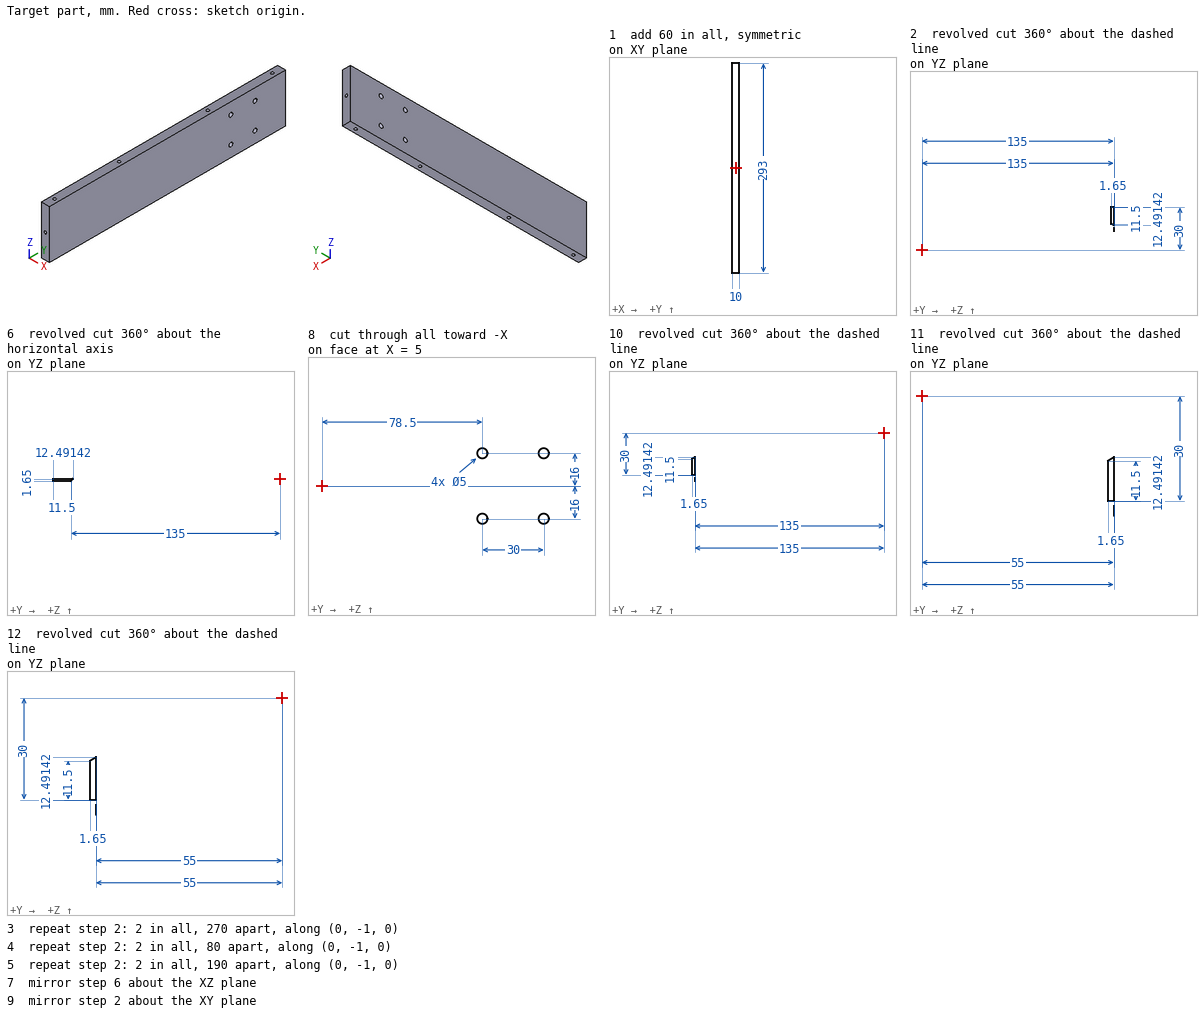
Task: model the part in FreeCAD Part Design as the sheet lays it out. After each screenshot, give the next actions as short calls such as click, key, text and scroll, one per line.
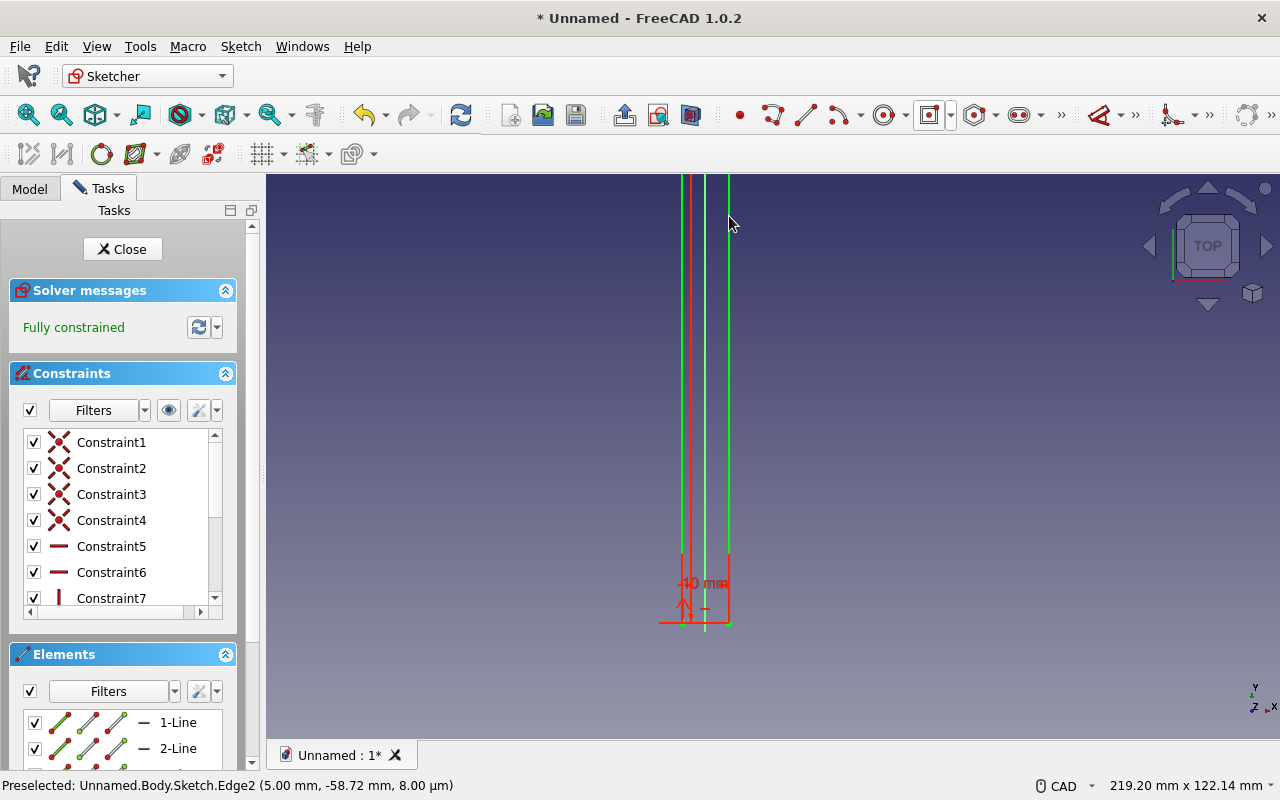
click(123, 249)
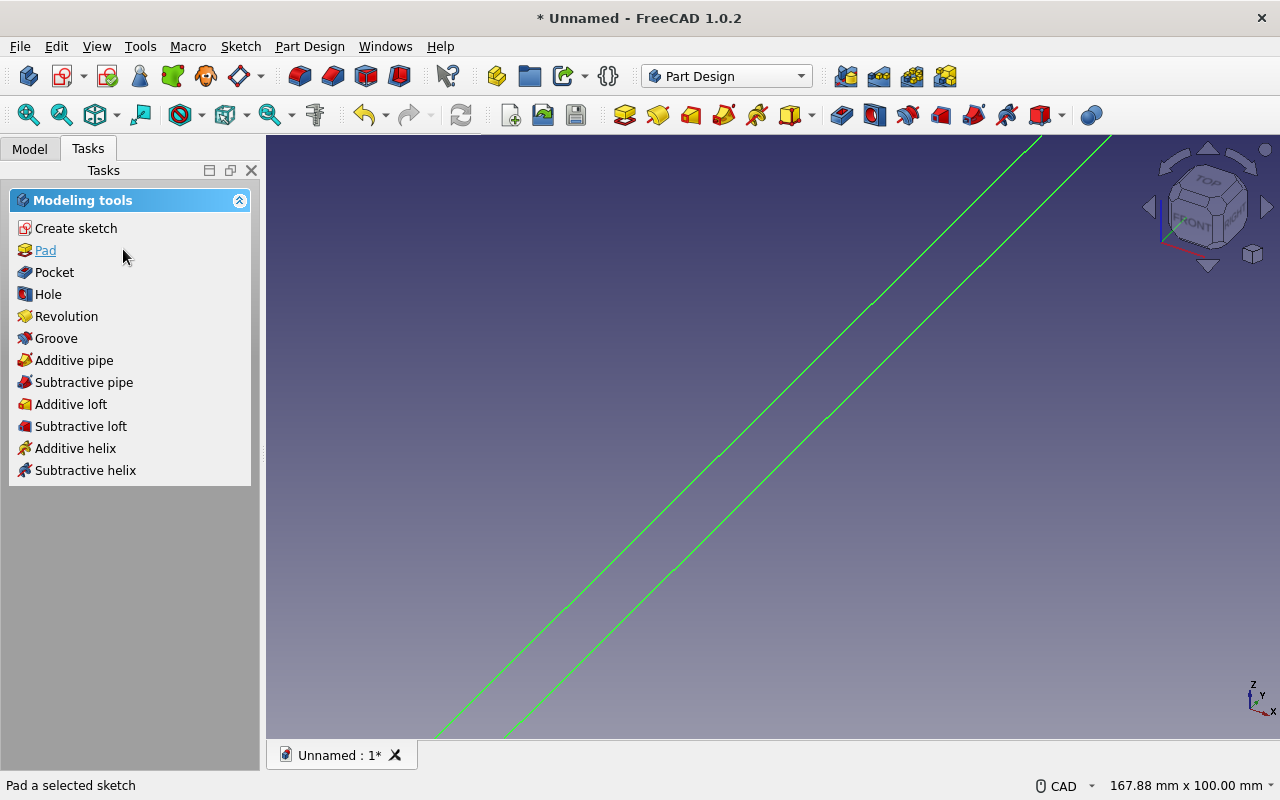
click(625, 116)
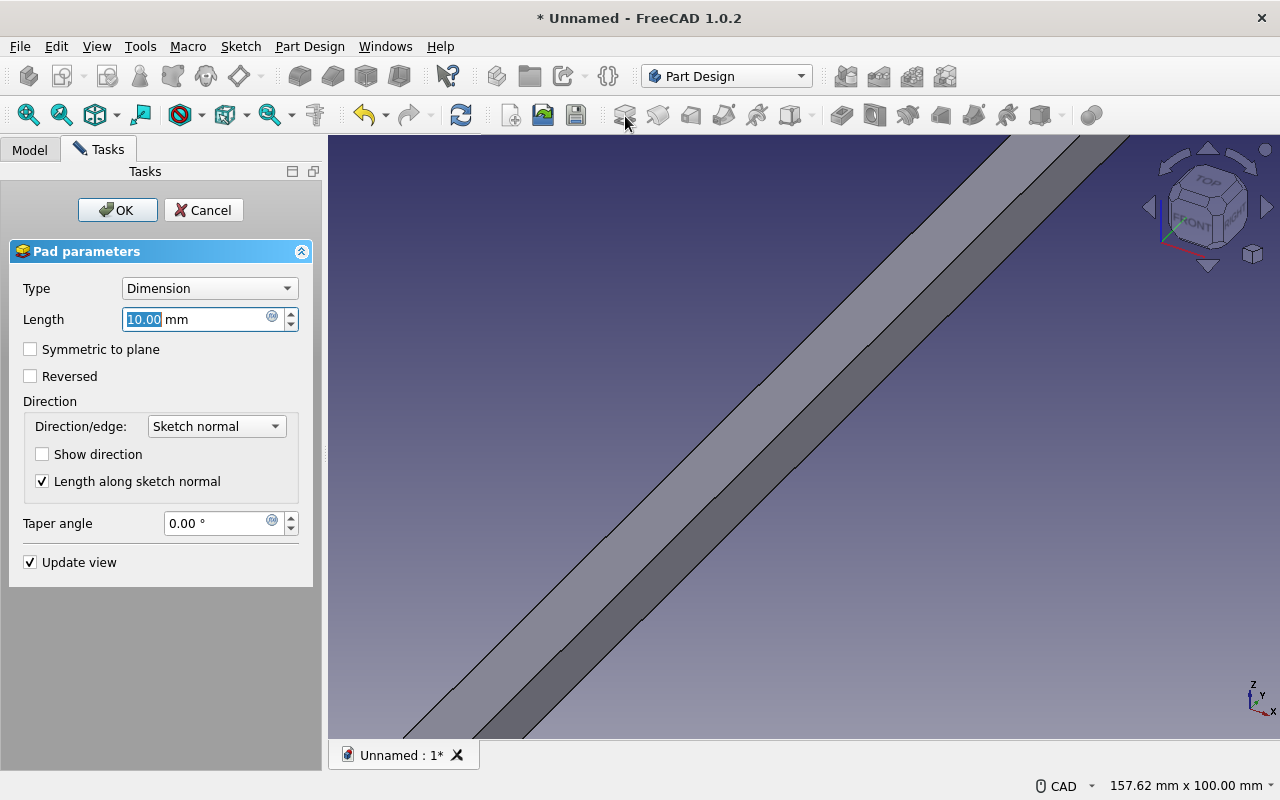
text(60)
key(Tab)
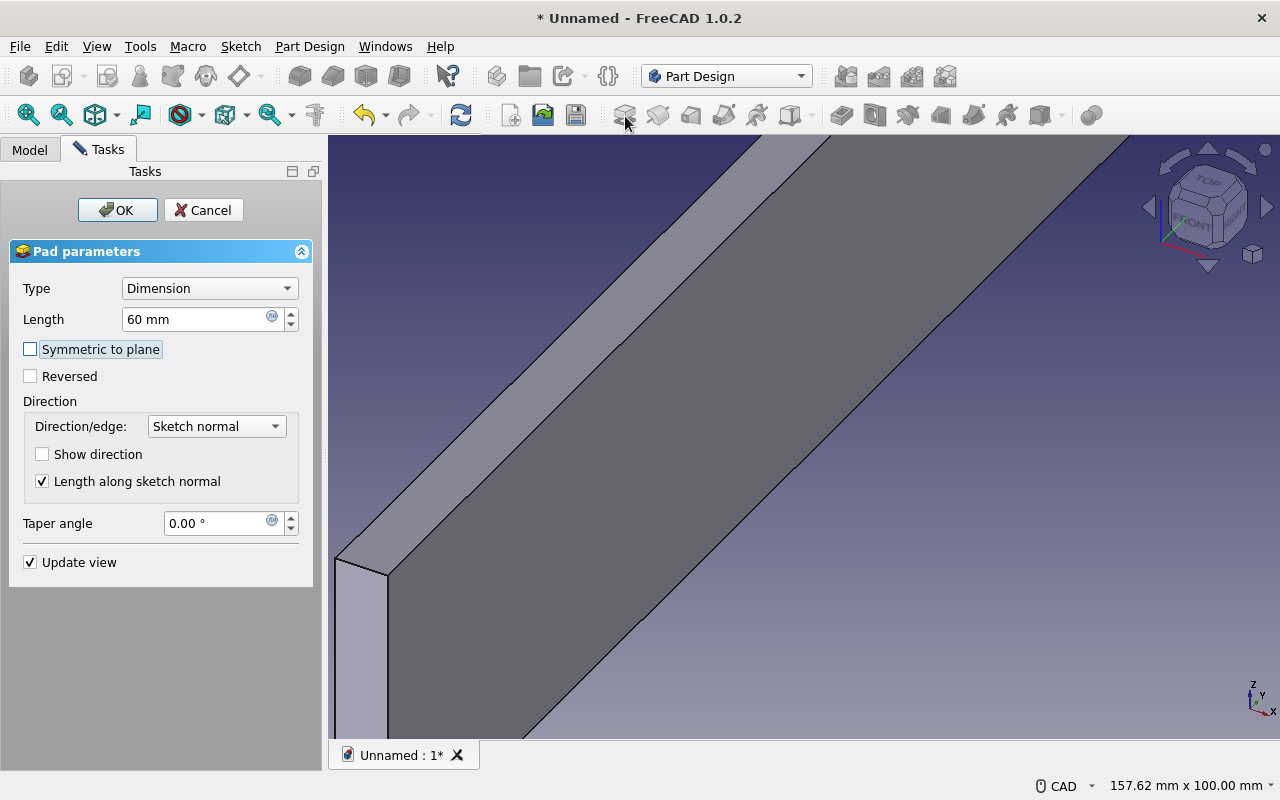
click(31, 349)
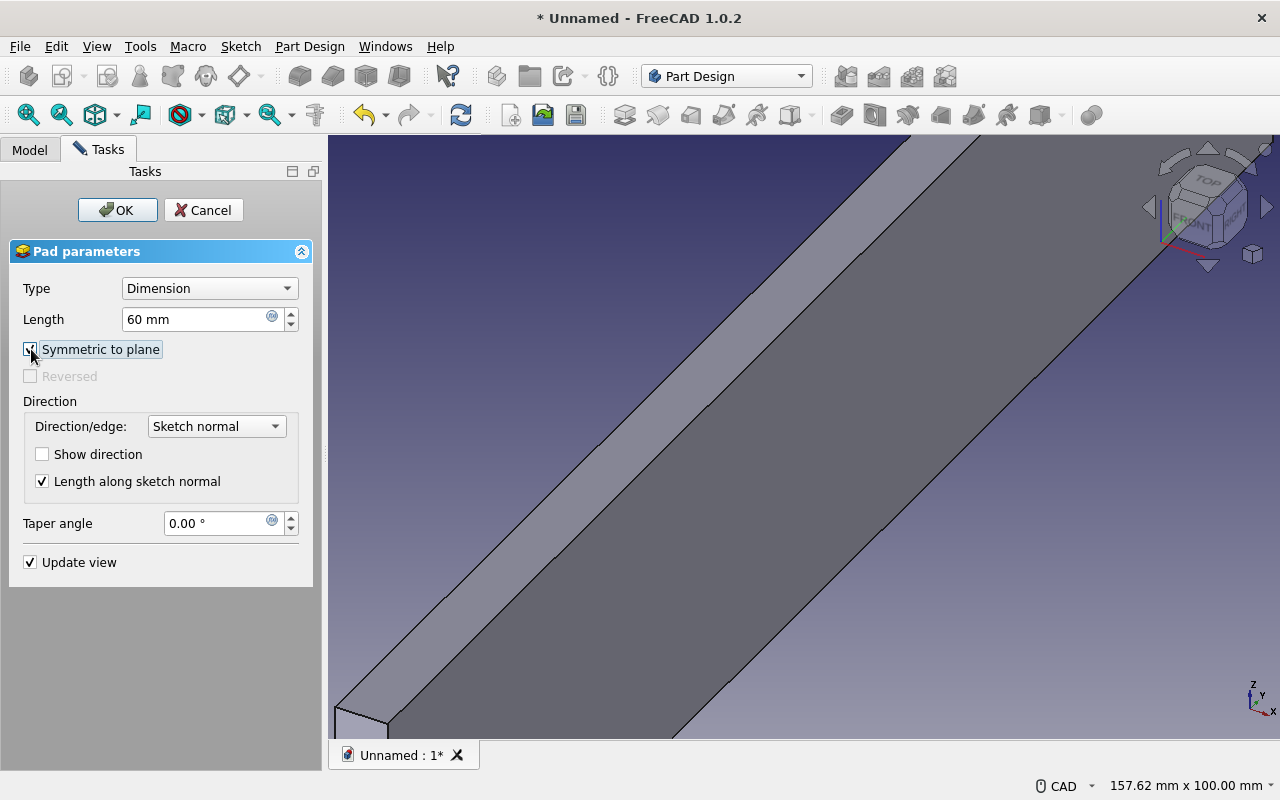
click(118, 210)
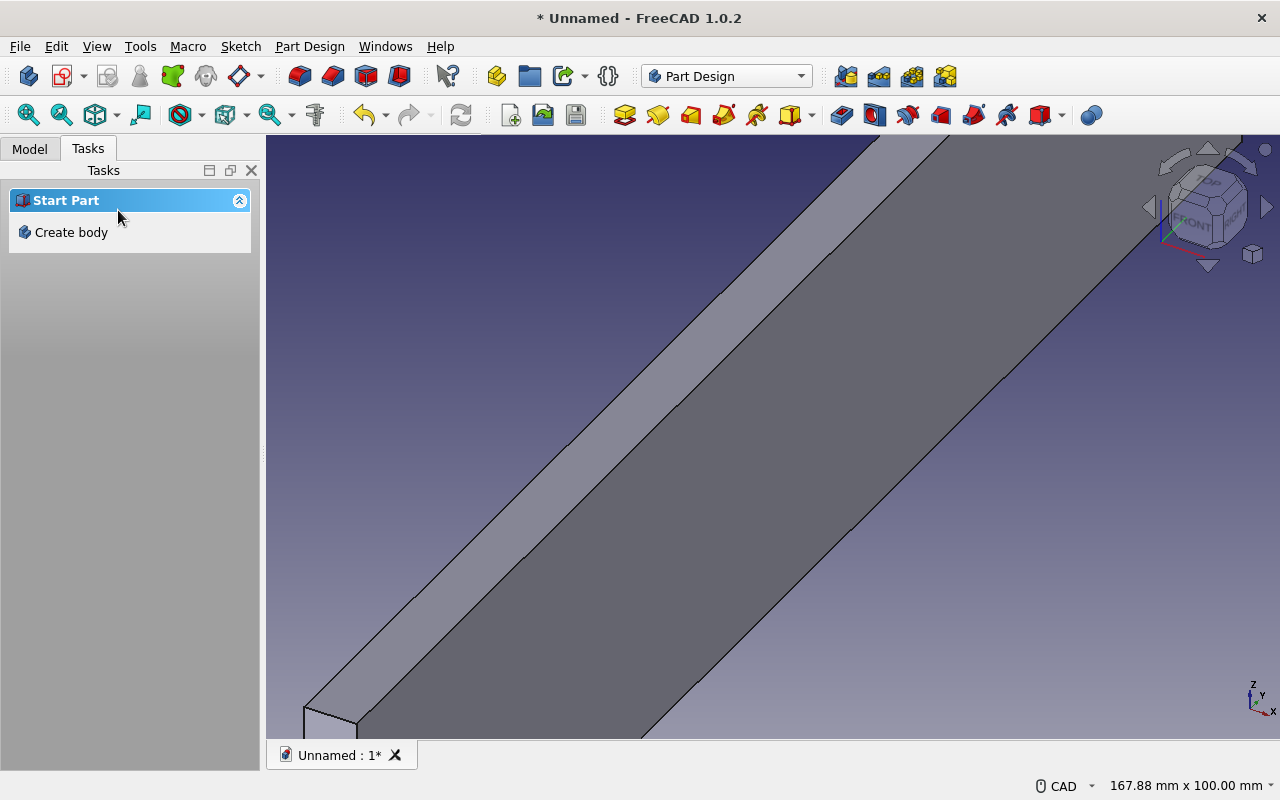
click(29, 116)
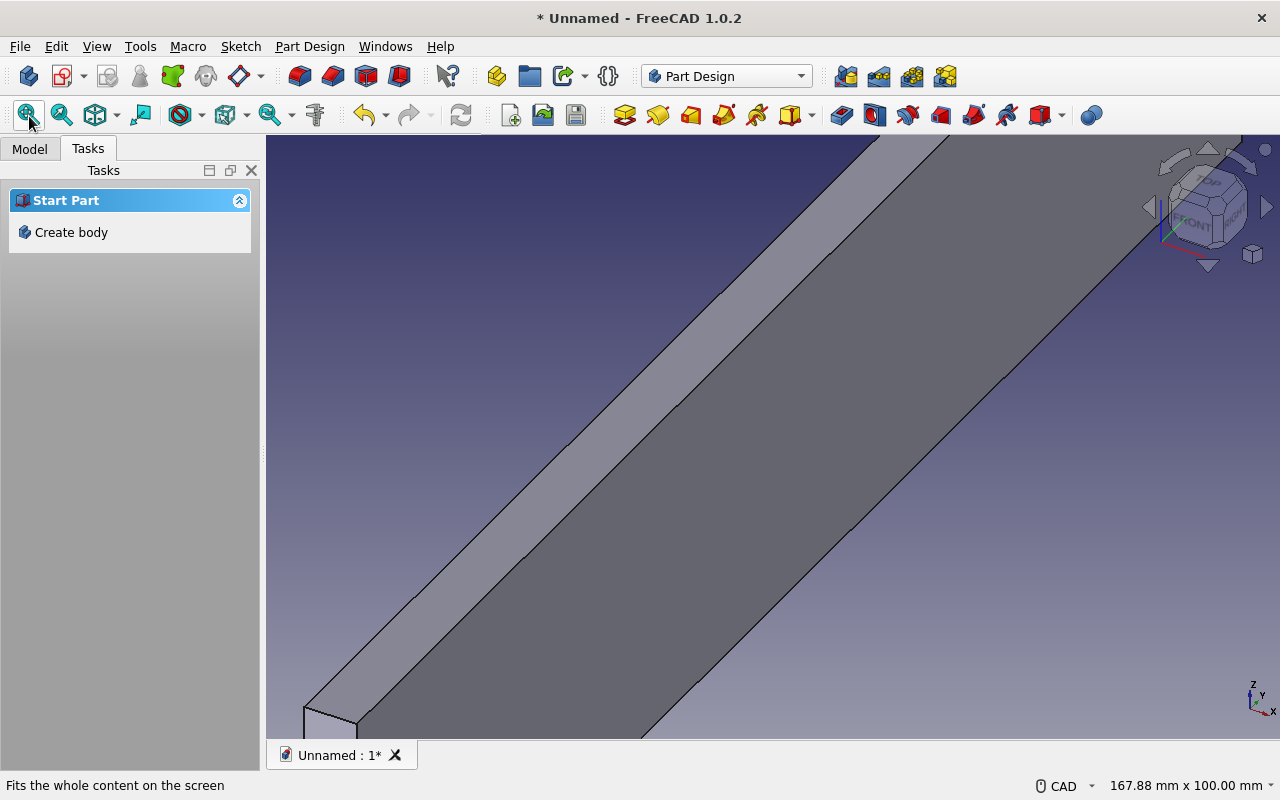
click(62, 76)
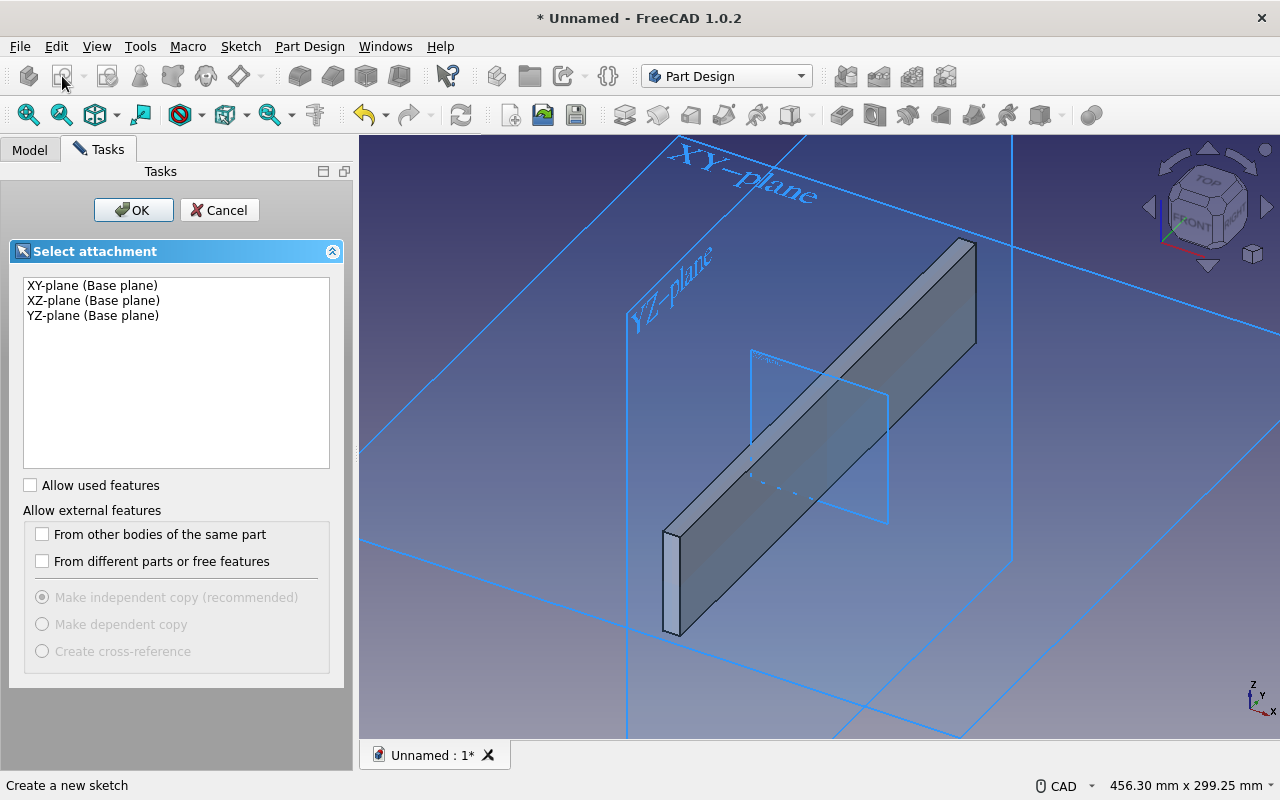
click(84, 316)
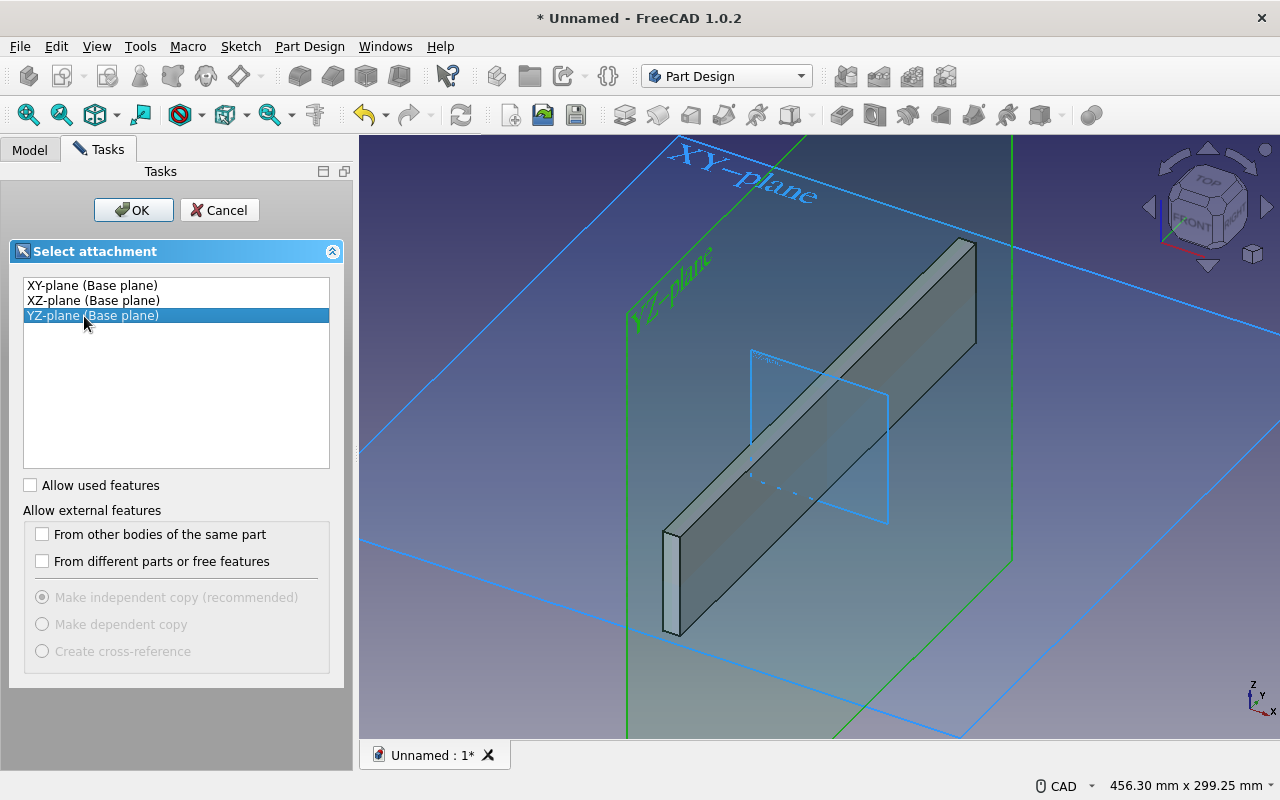
click(134, 210)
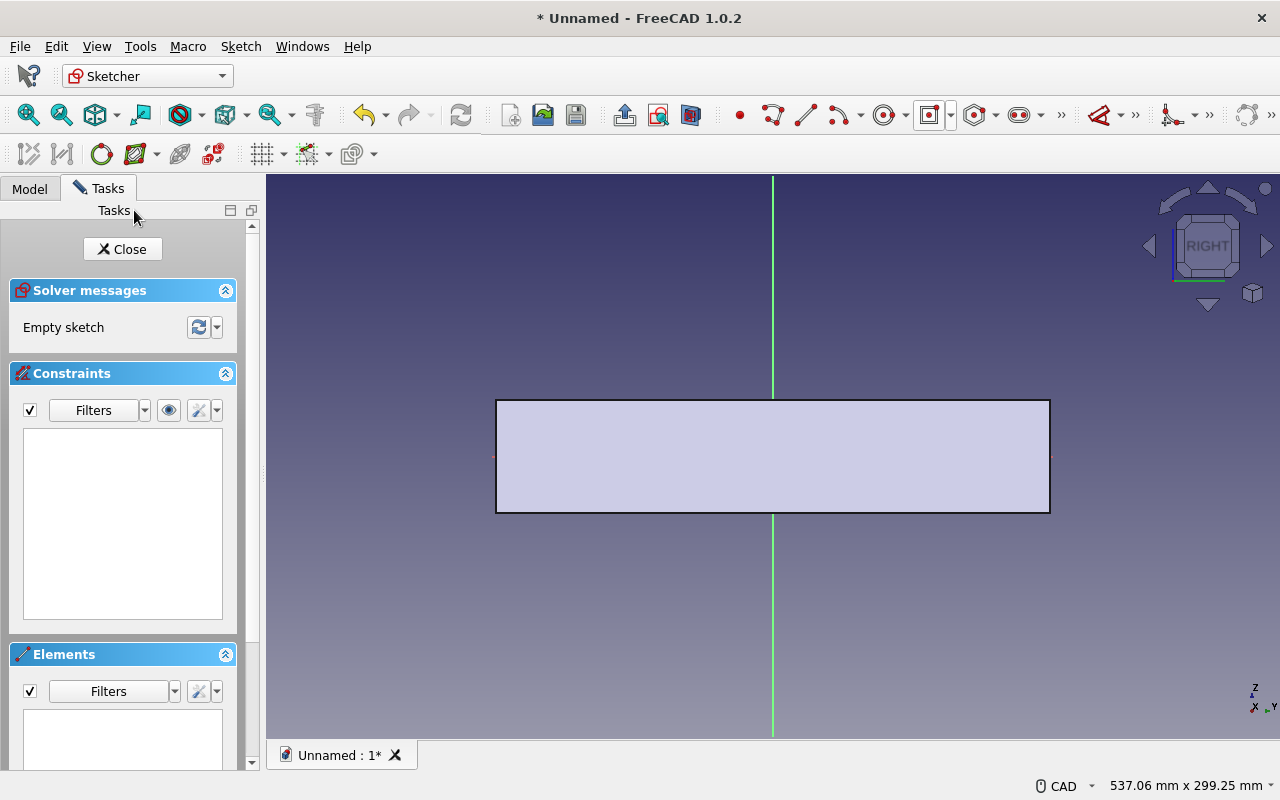
click(691, 116)